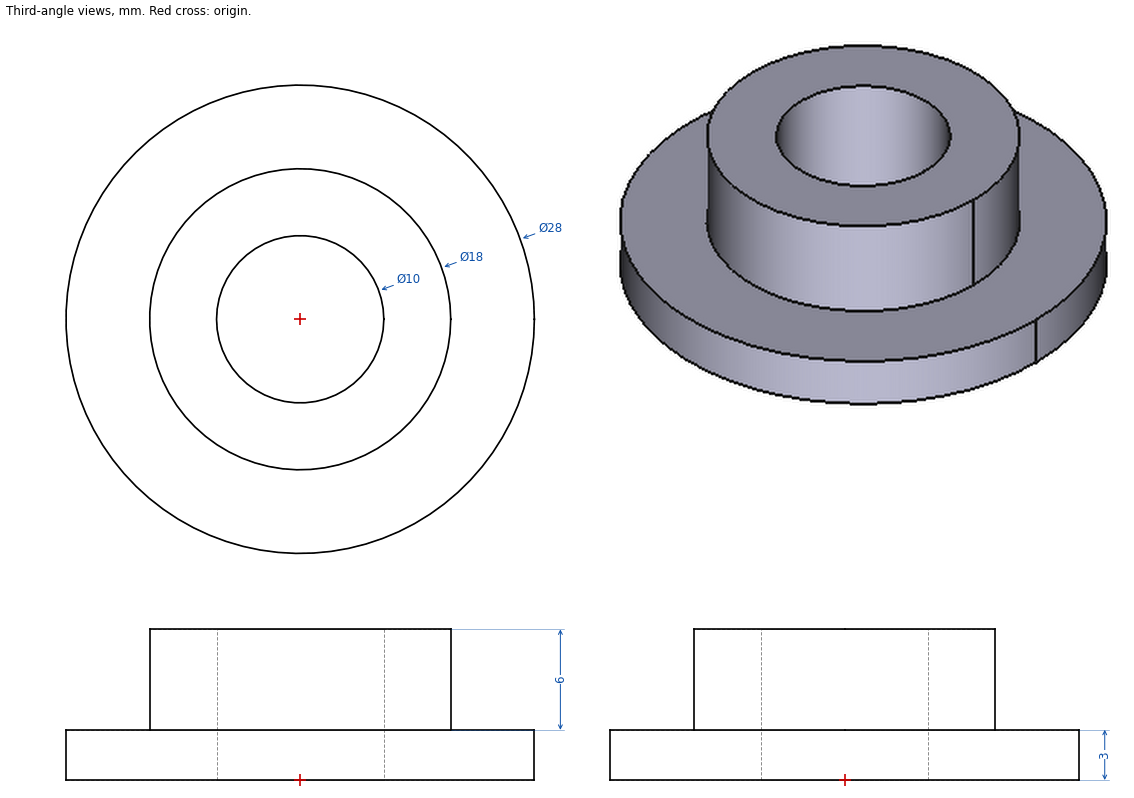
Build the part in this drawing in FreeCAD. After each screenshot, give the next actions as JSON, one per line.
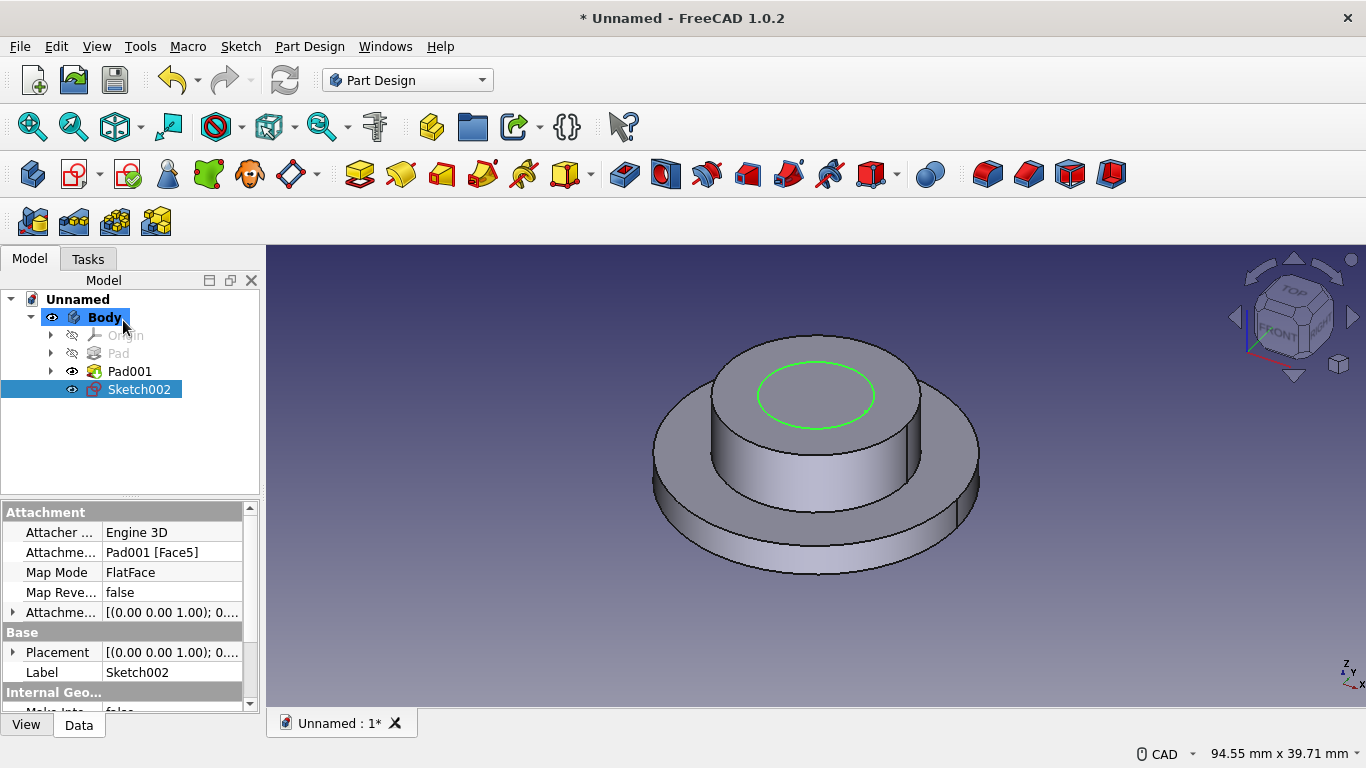
{"action": "left_click", "coordinate": [625, 174]}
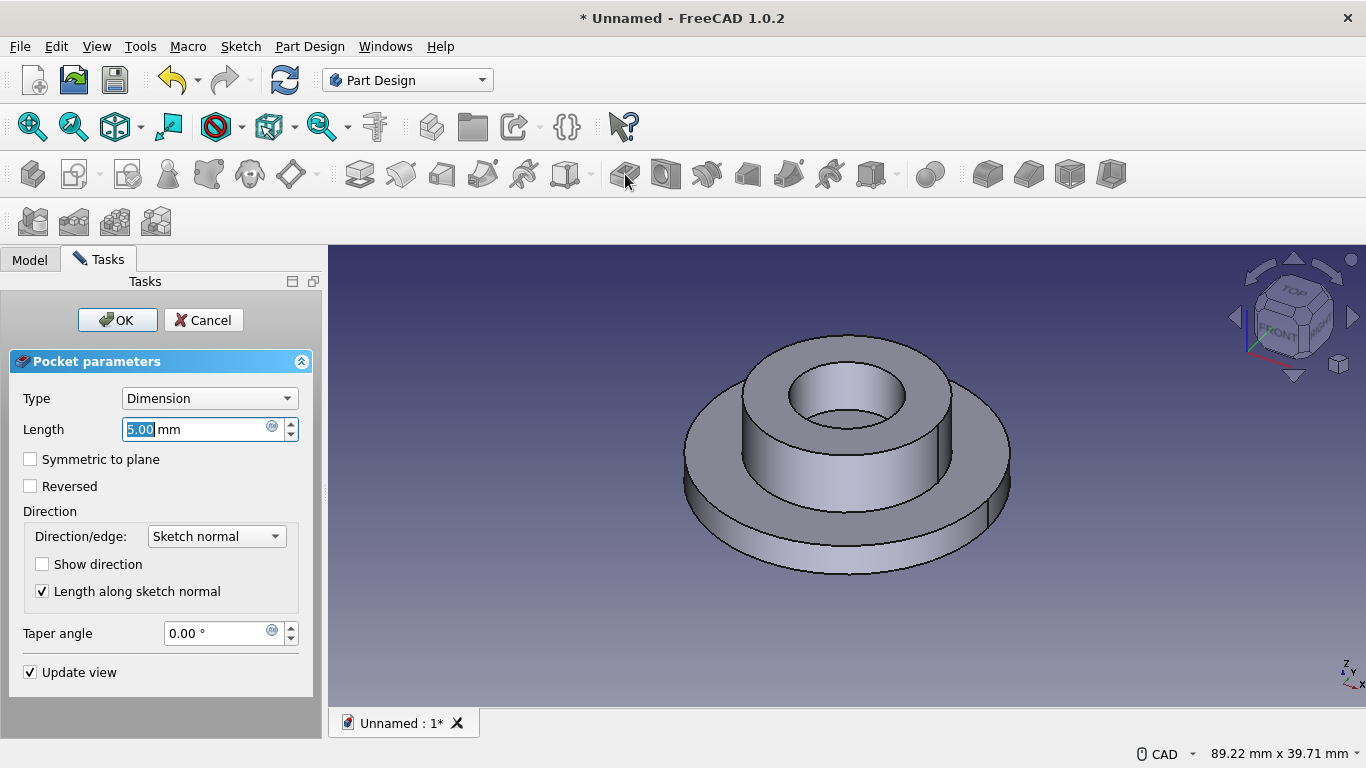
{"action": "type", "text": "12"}
{"action": "key", "text": "Tab"}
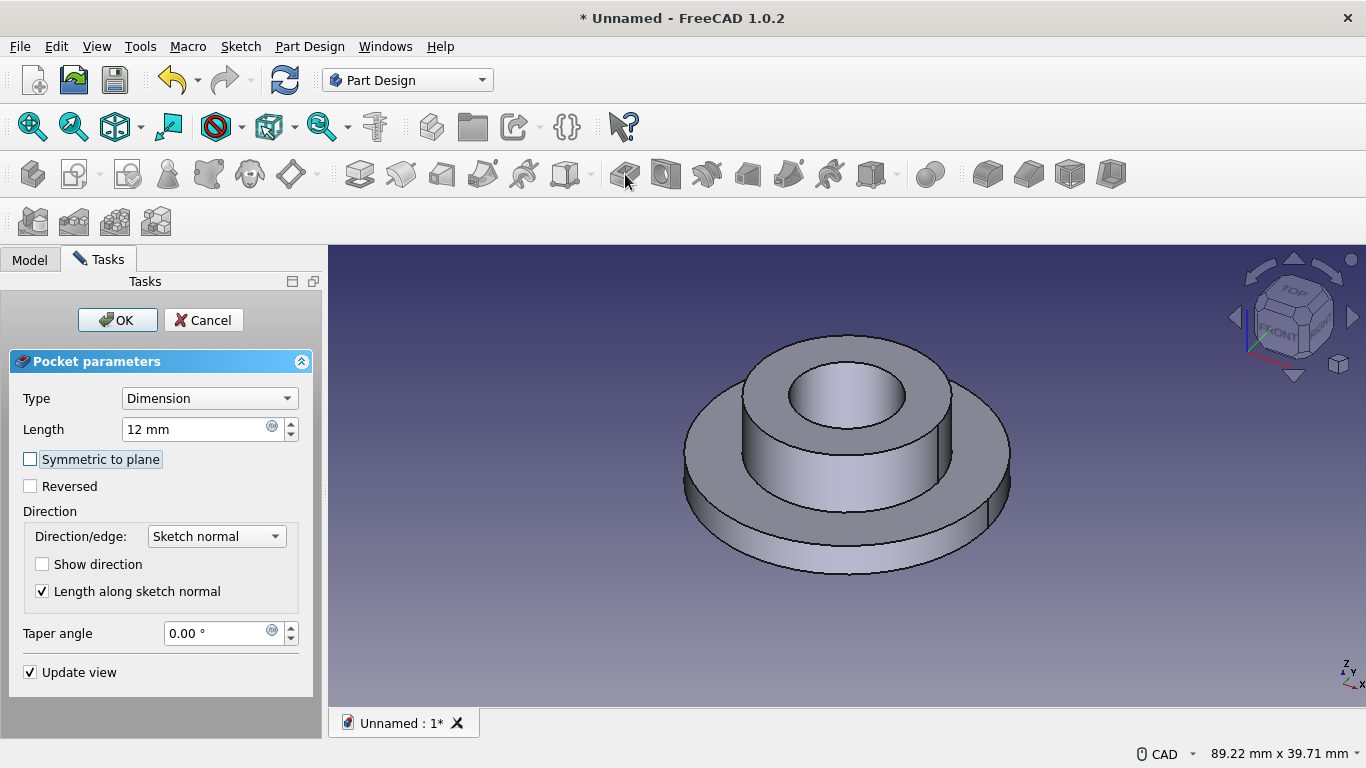
{"action": "left_click", "coordinate": [118, 320]}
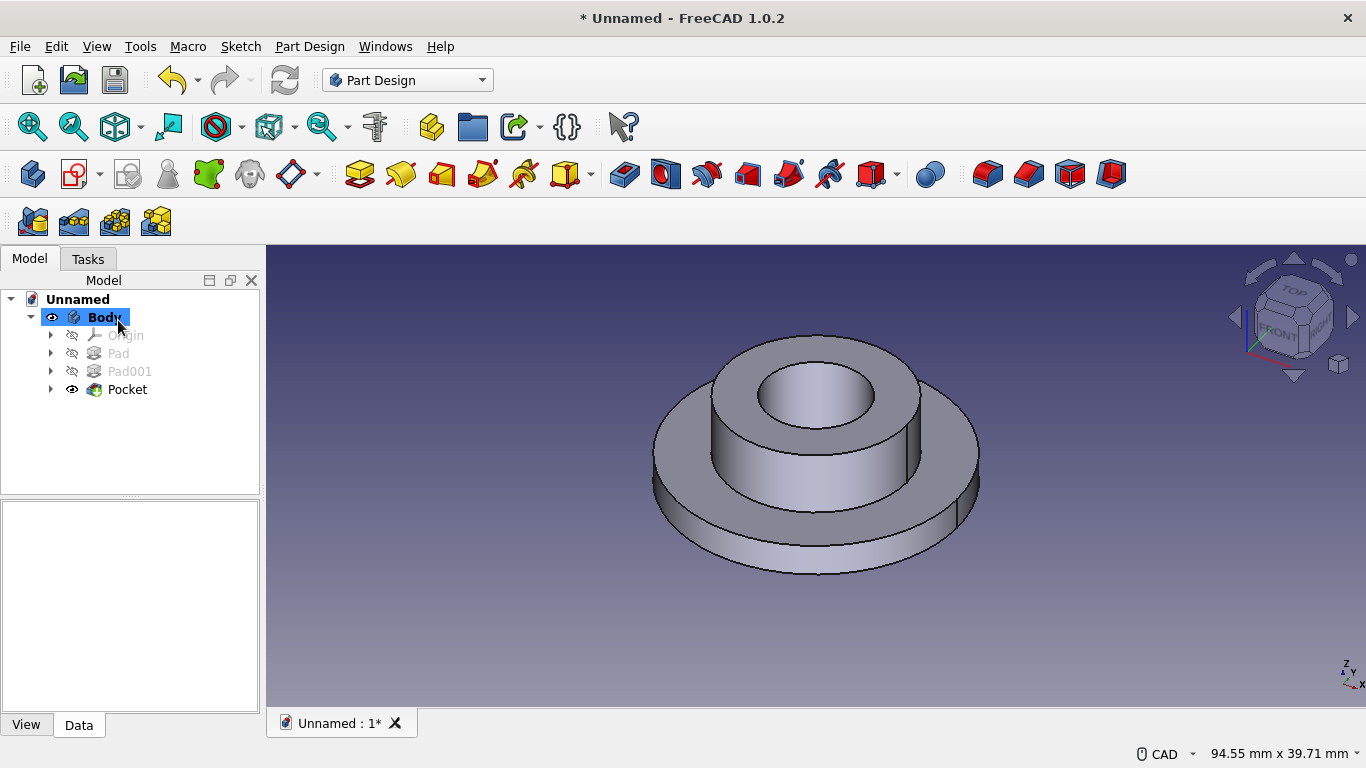
{"action": "key", "text": "0"}